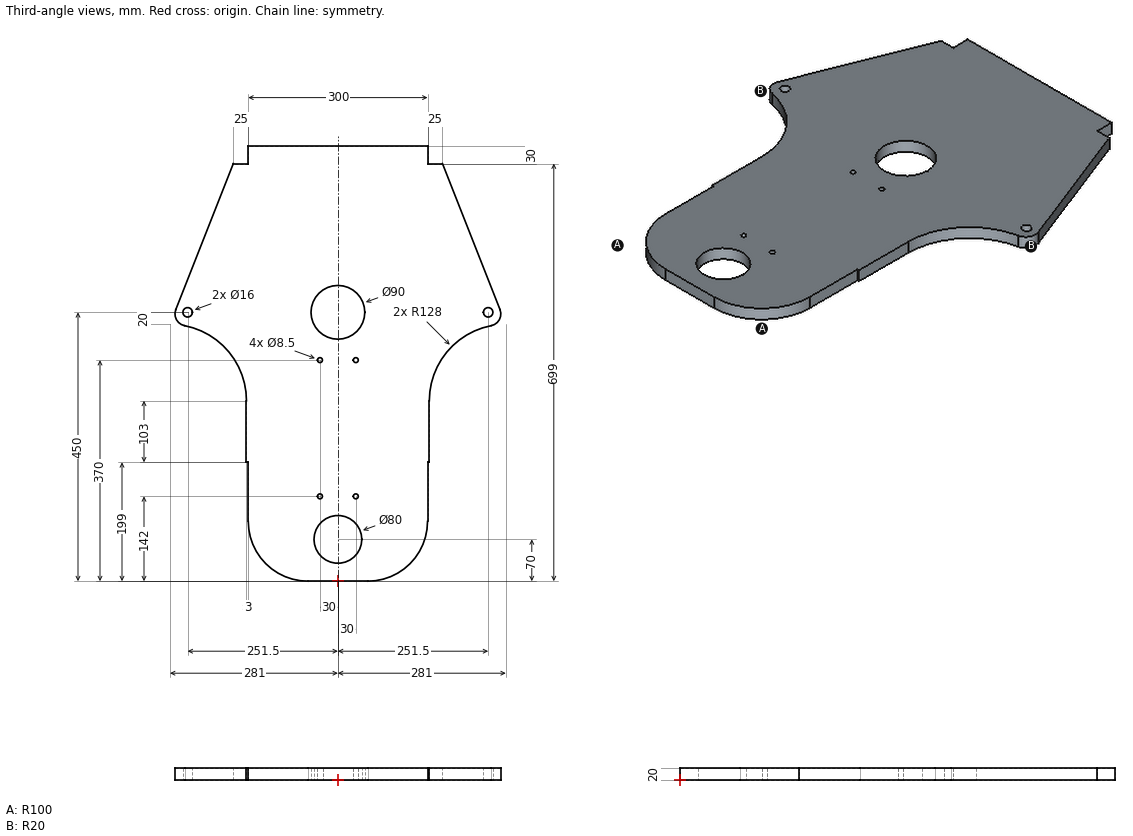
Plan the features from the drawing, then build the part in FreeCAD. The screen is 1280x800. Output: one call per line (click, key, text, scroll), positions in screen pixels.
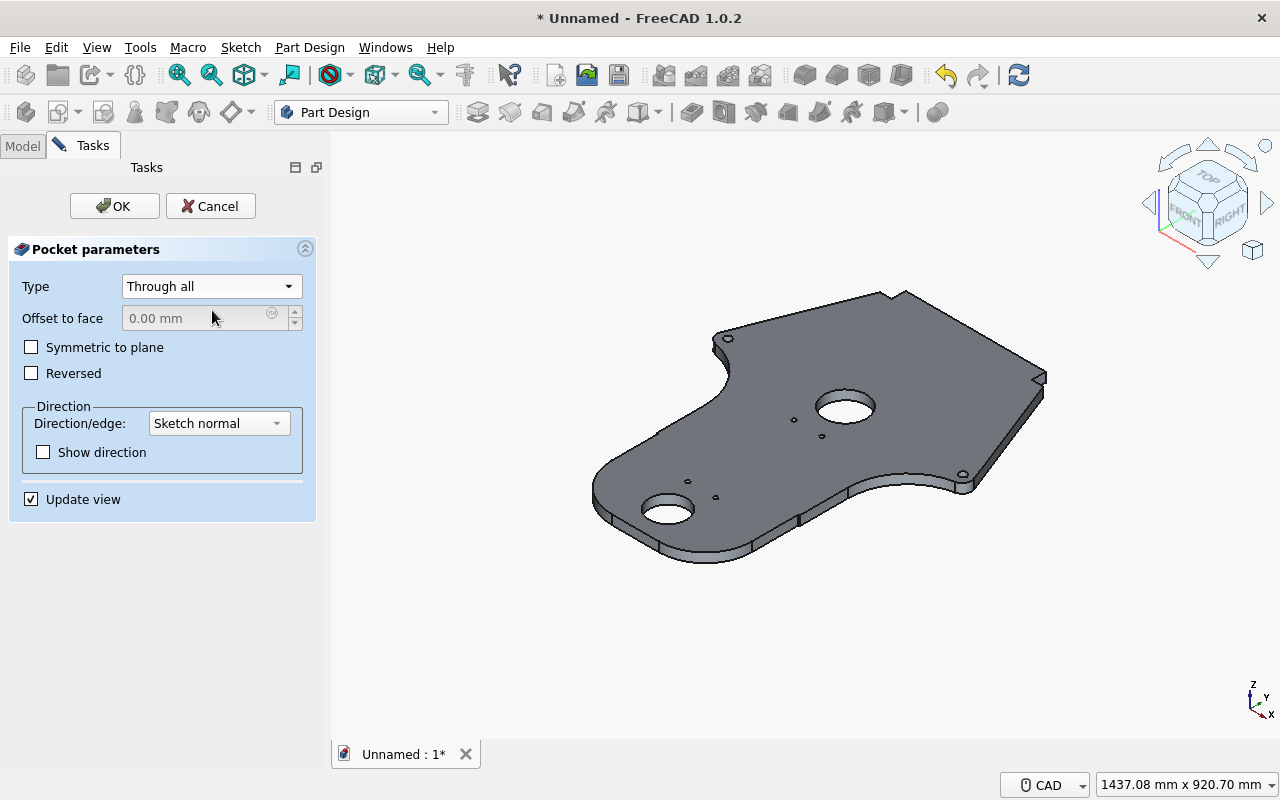
click(115, 206)